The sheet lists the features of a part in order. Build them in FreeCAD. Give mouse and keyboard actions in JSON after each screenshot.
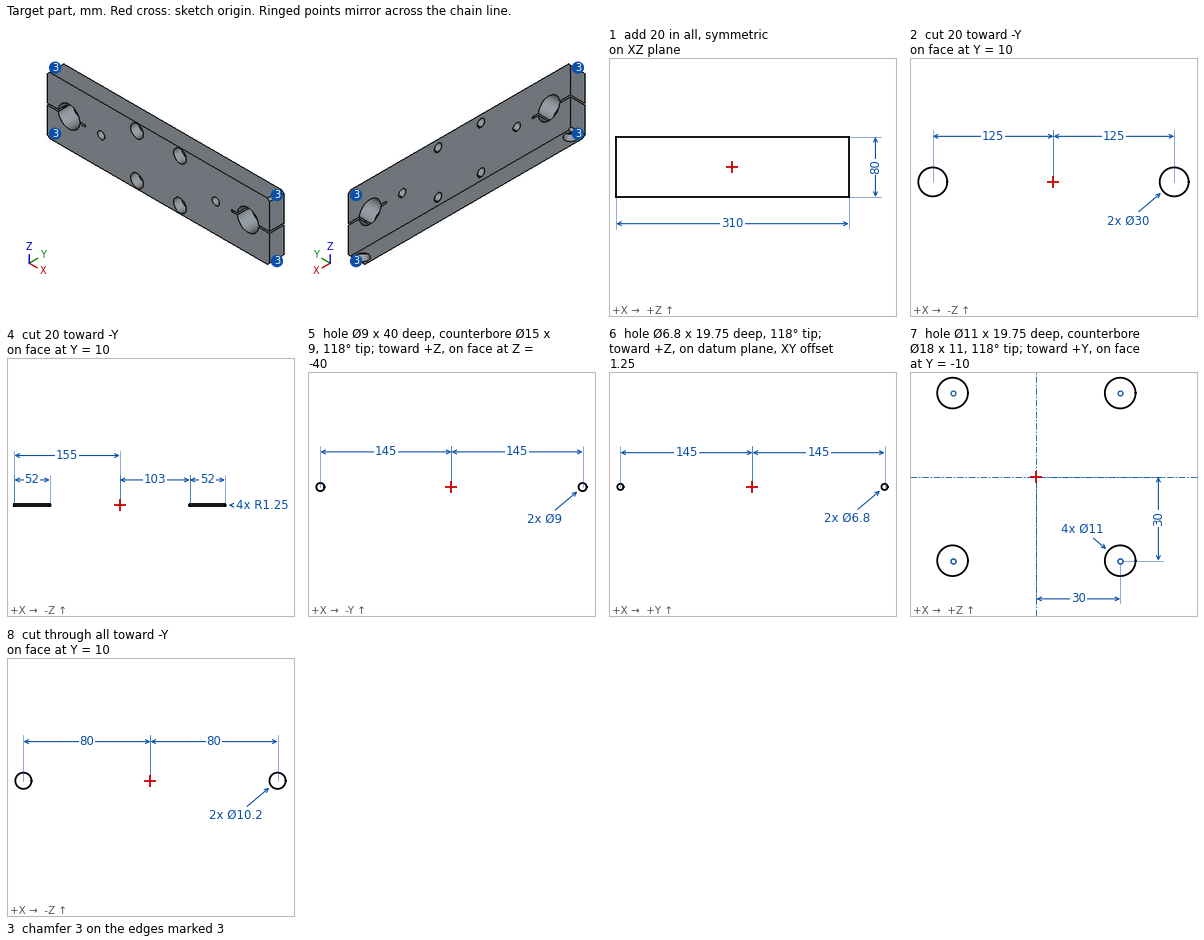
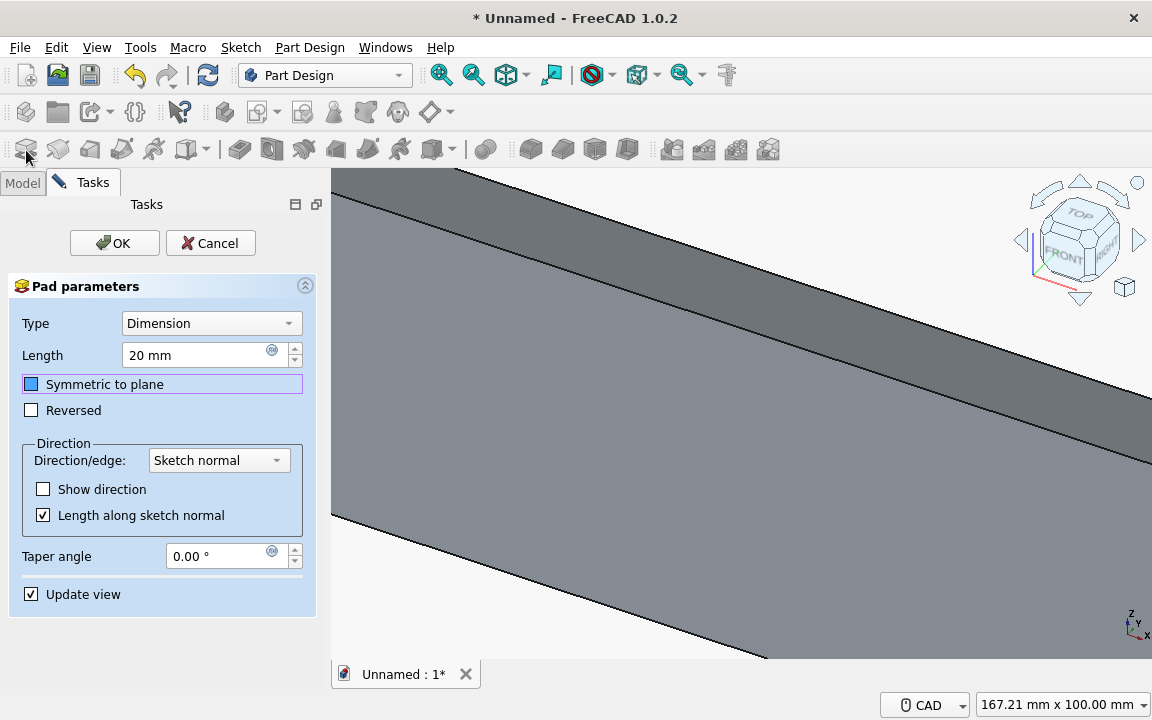
{"action": "left_click", "coordinate": [30, 384]}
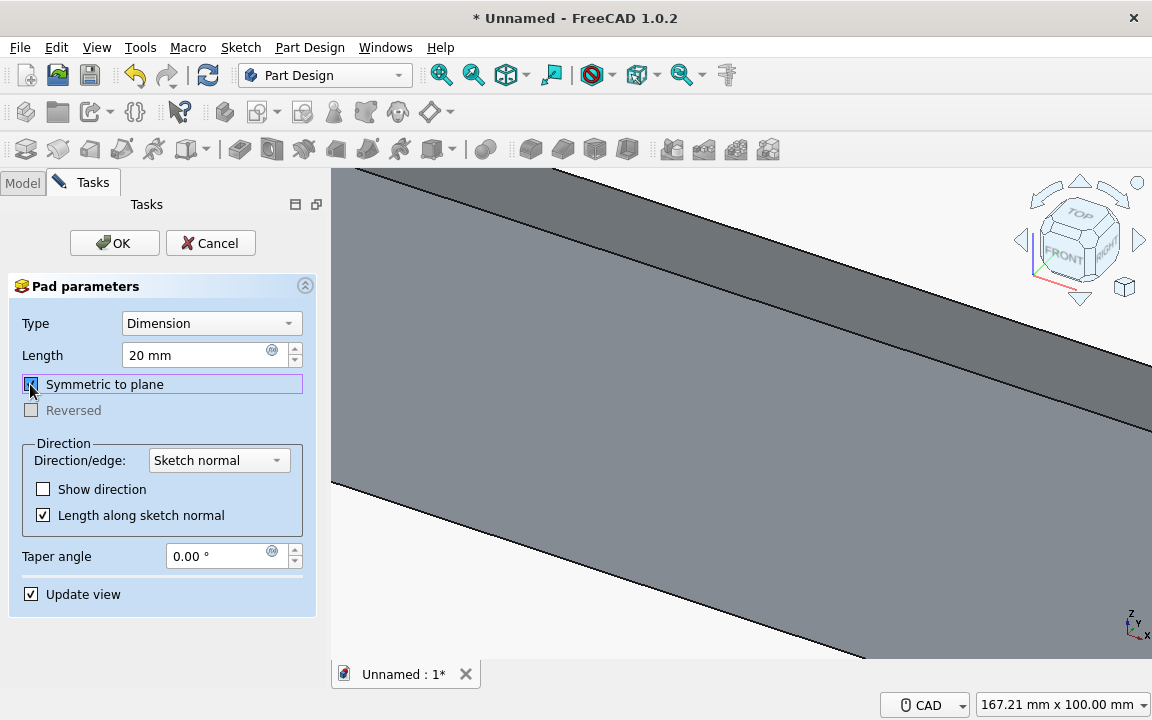
{"action": "left_click", "coordinate": [115, 243]}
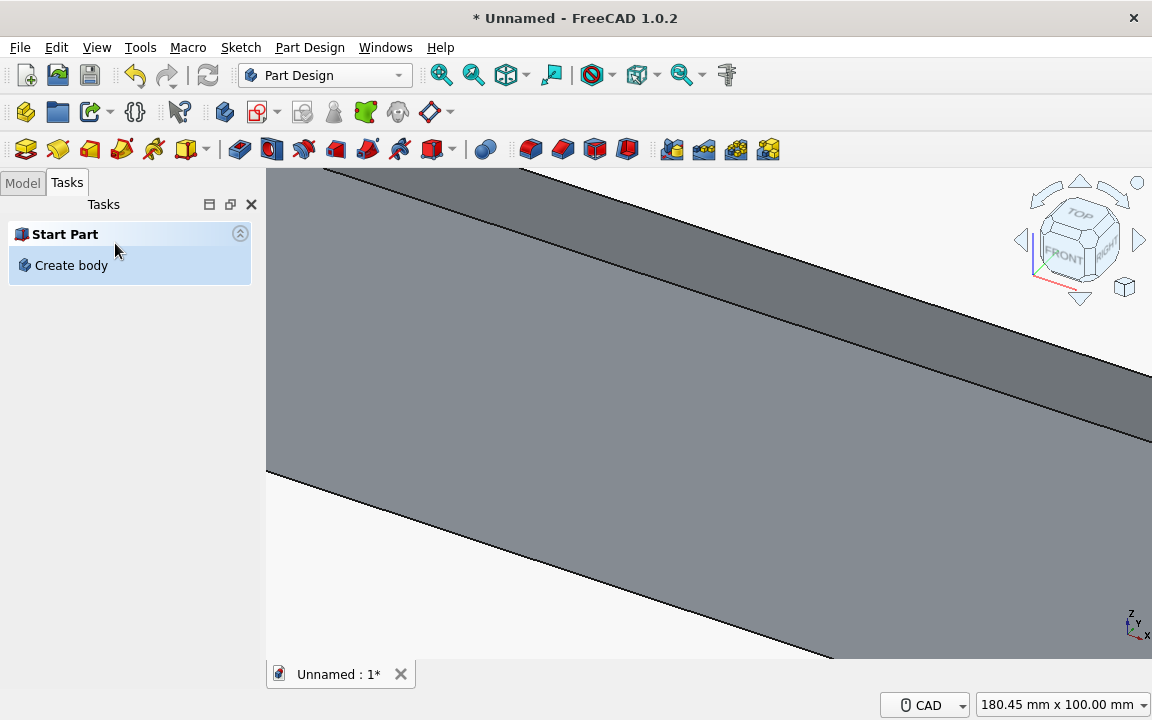
{"action": "left_click", "coordinate": [442, 76]}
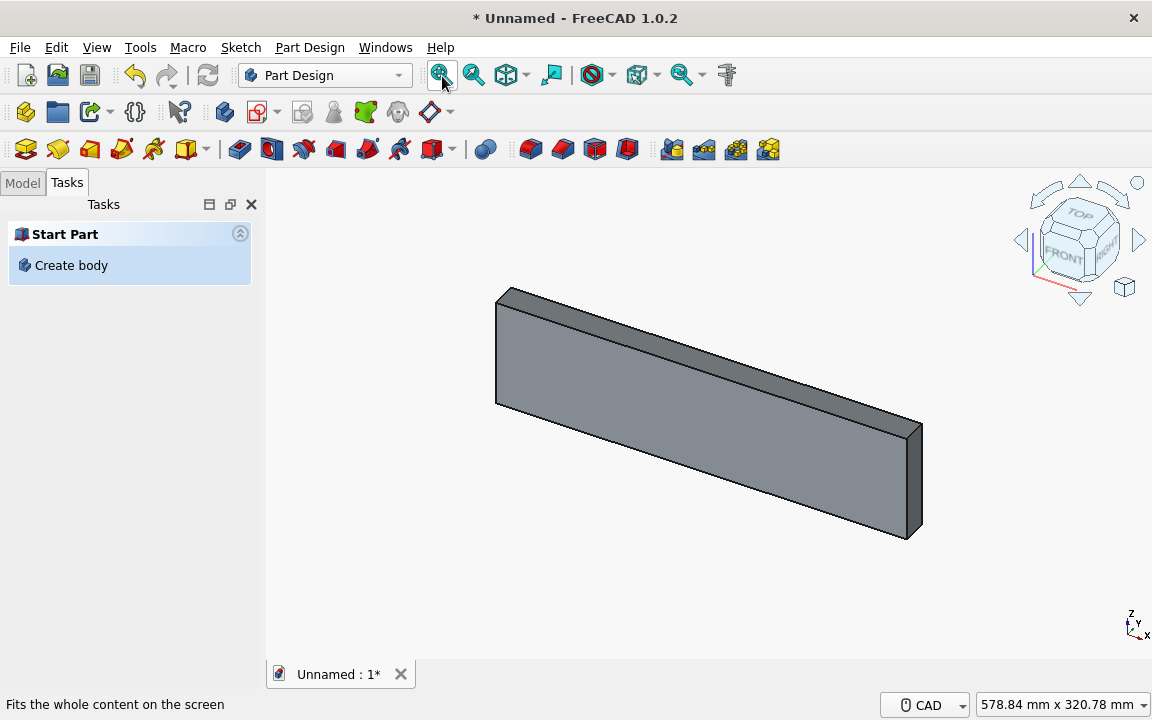
{"action": "key", "text": "4"}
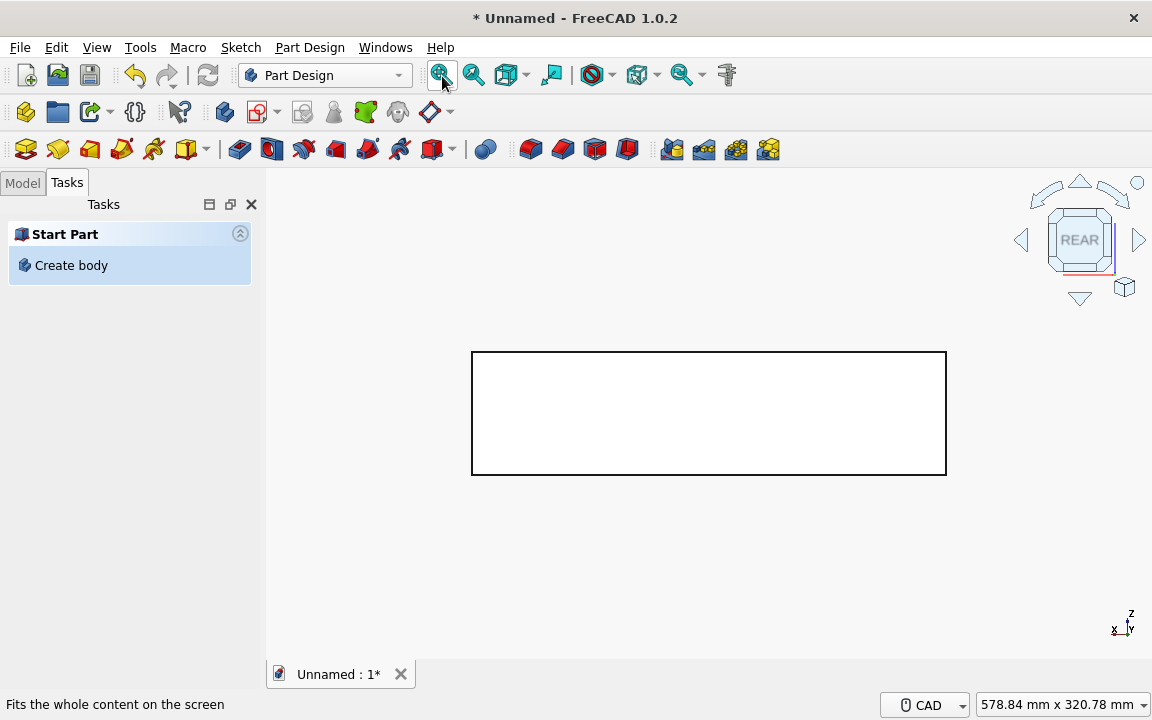
{"action": "left_click", "coordinate": [573, 412]}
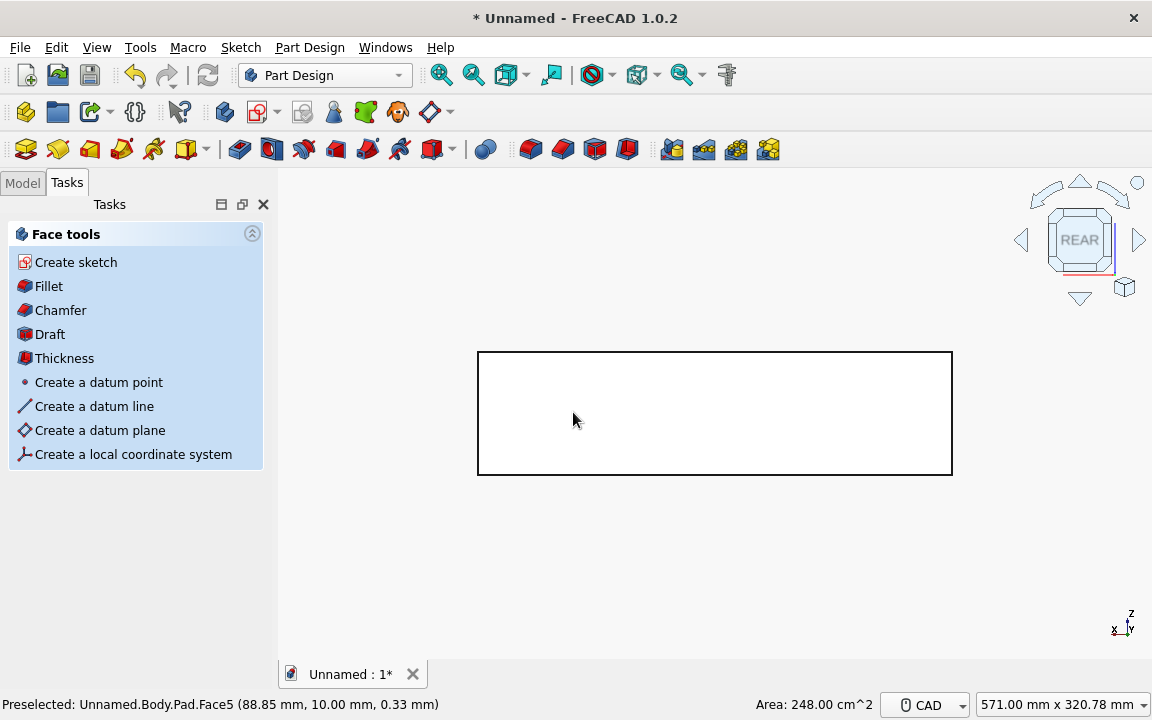
{"action": "left_click", "coordinate": [258, 112]}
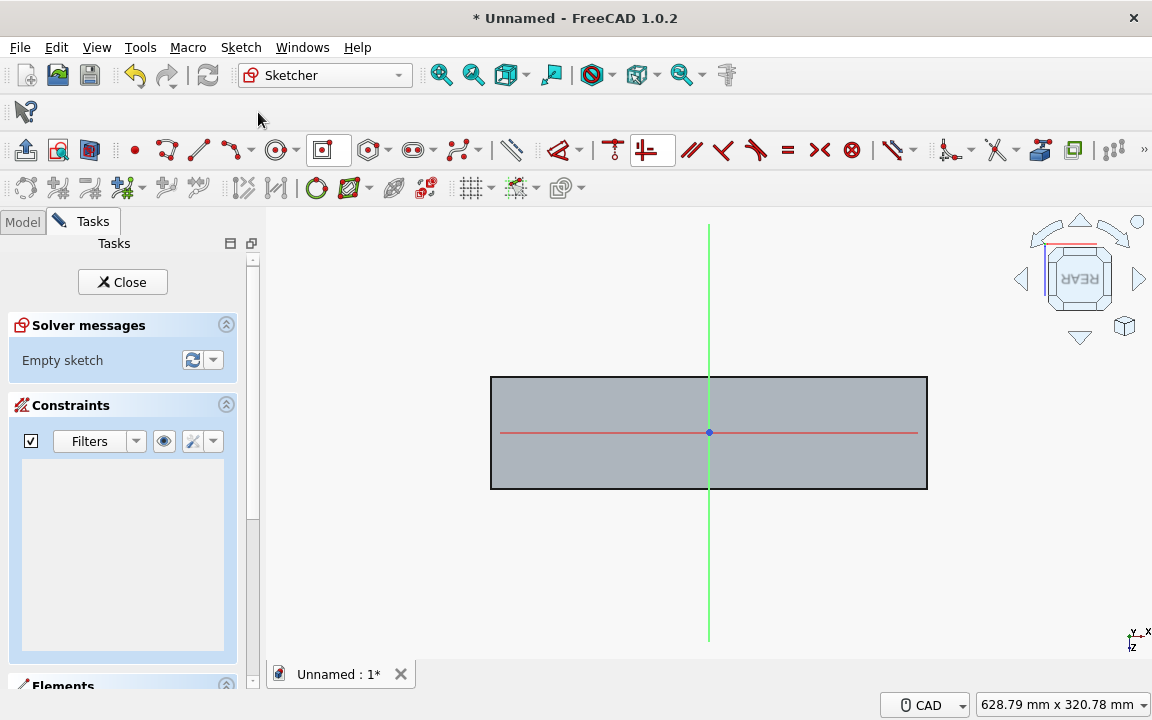
{"action": "left_click", "coordinate": [276, 150]}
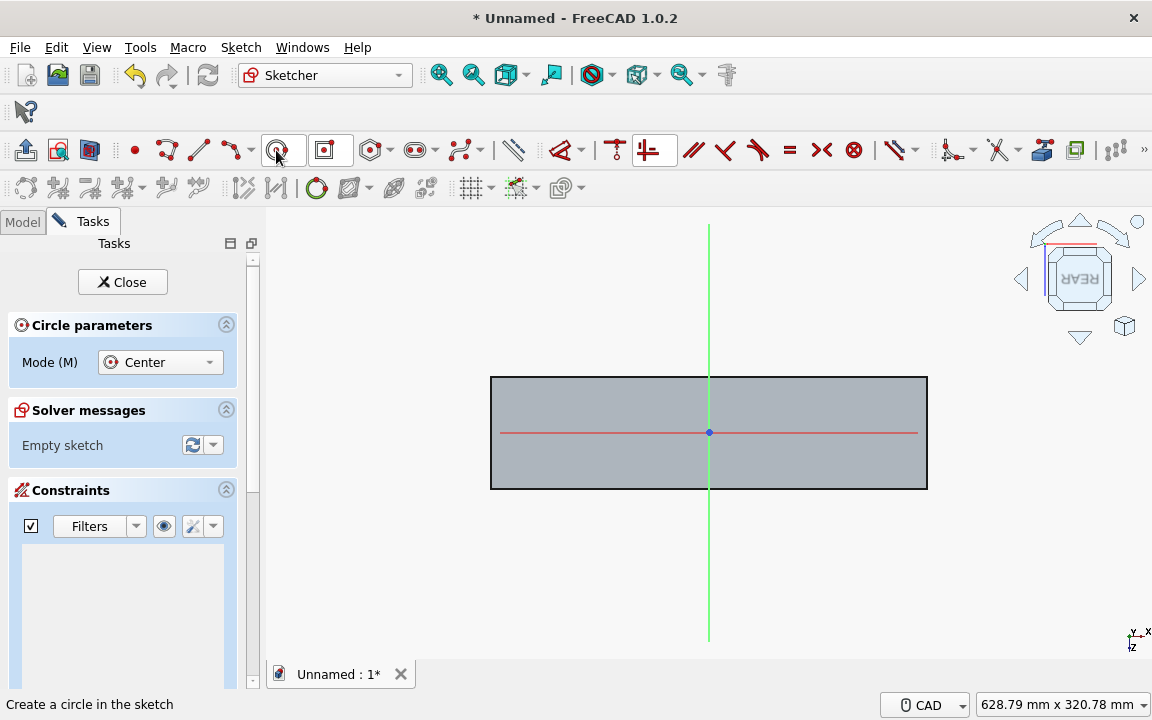
{"action": "left_click", "coordinate": [885, 433]}
{"action": "mouse_move", "coordinate": [900, 418]}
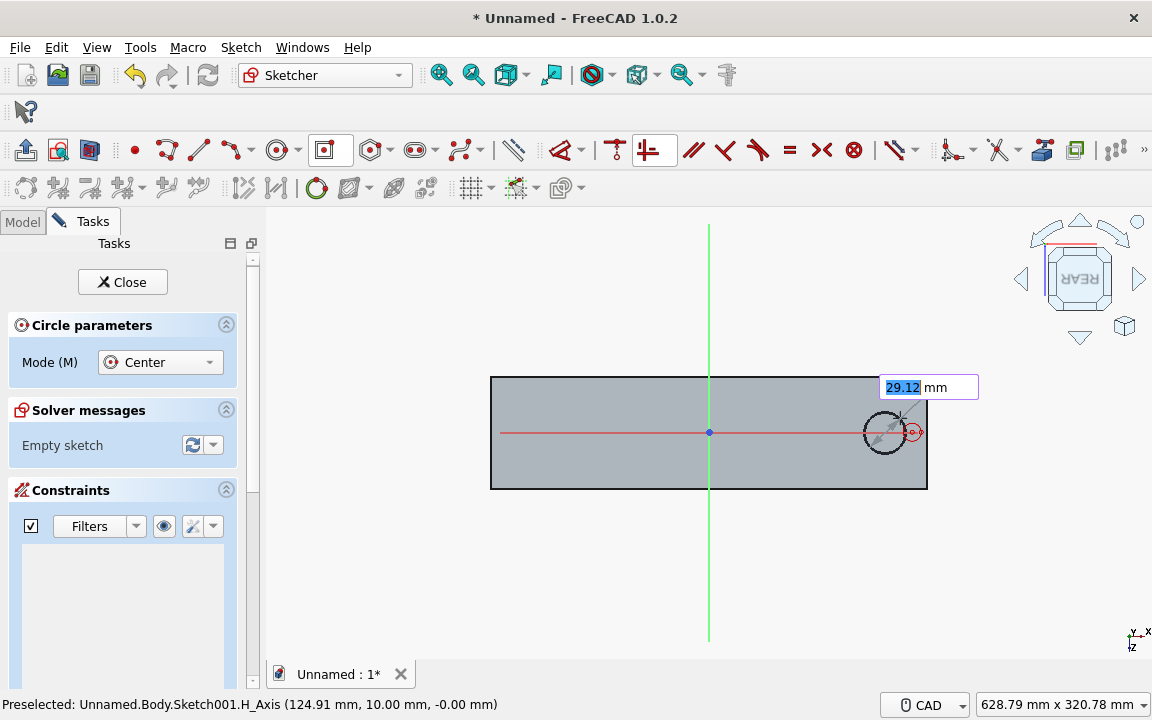
{"action": "type", "text": "30"}
{"action": "key", "text": "Return"}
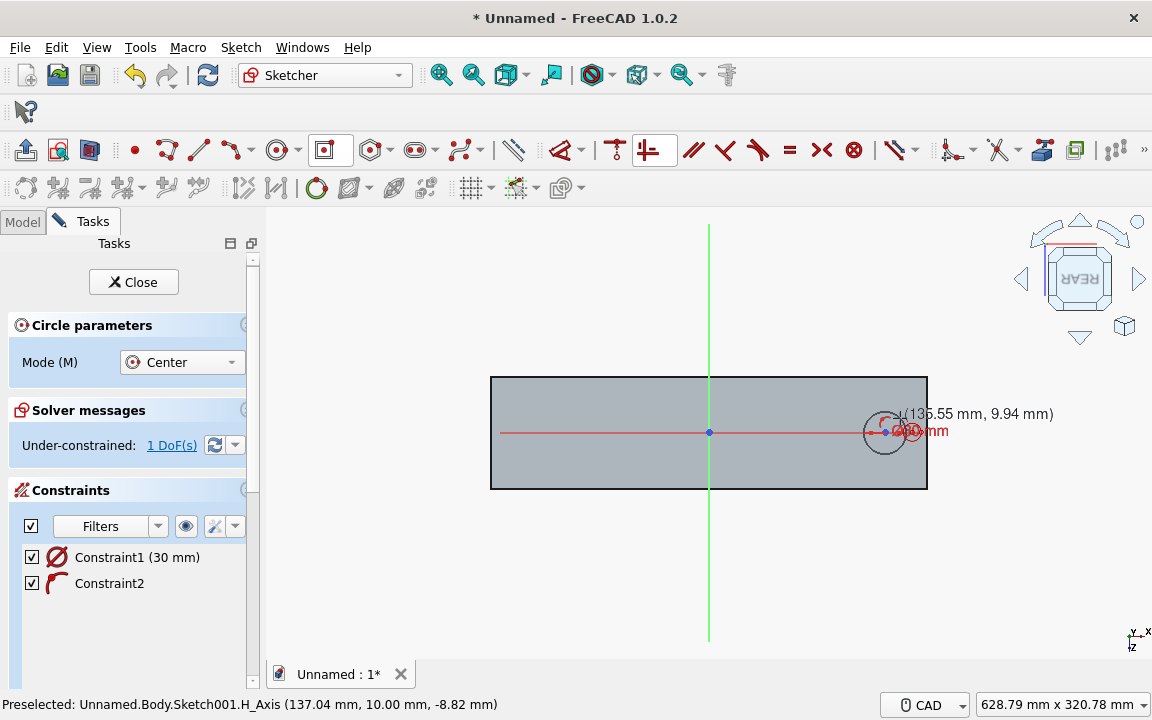
{"action": "left_click", "coordinate": [533, 433]}
{"action": "mouse_move", "coordinate": [548, 418]}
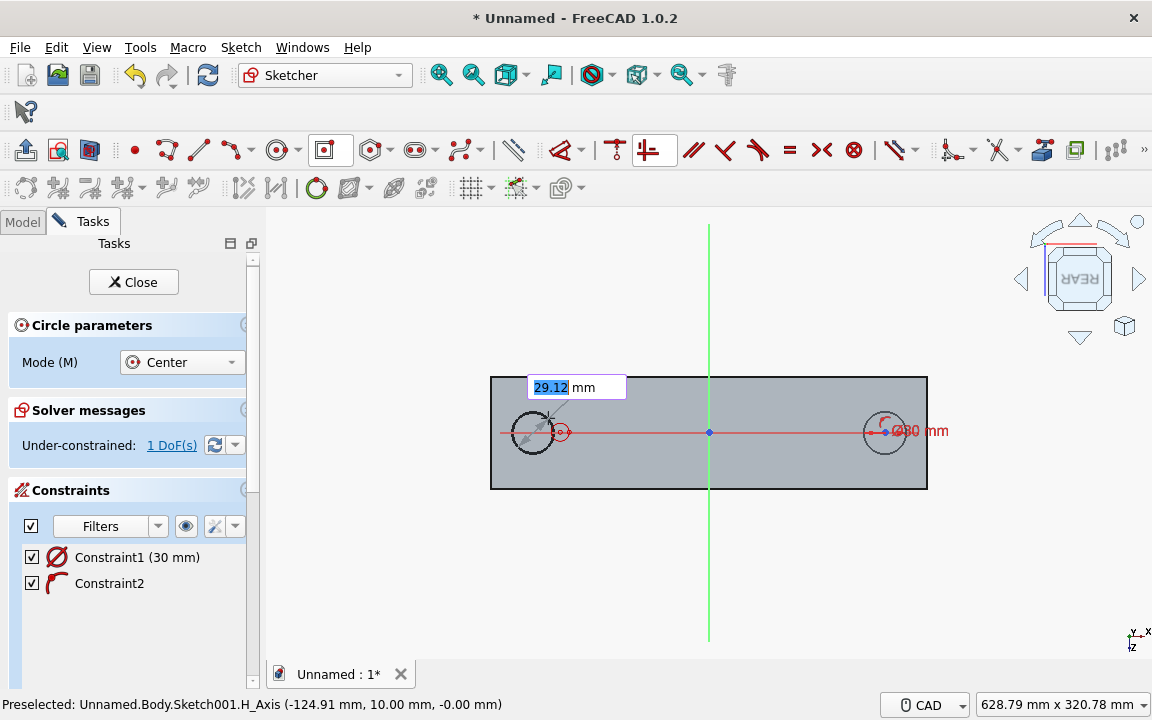
{"action": "type", "text": "30"}
{"action": "key", "text": "Return"}
{"action": "key", "text": "Escape"}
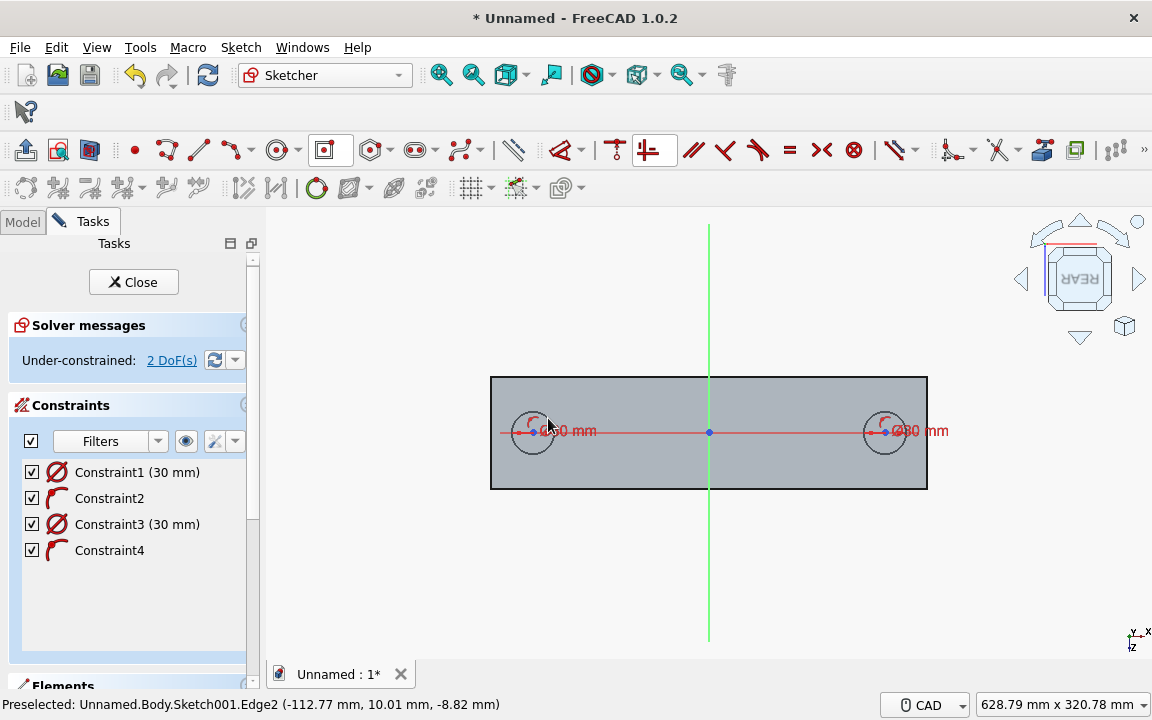
{"action": "left_click", "coordinate": [560, 150]}